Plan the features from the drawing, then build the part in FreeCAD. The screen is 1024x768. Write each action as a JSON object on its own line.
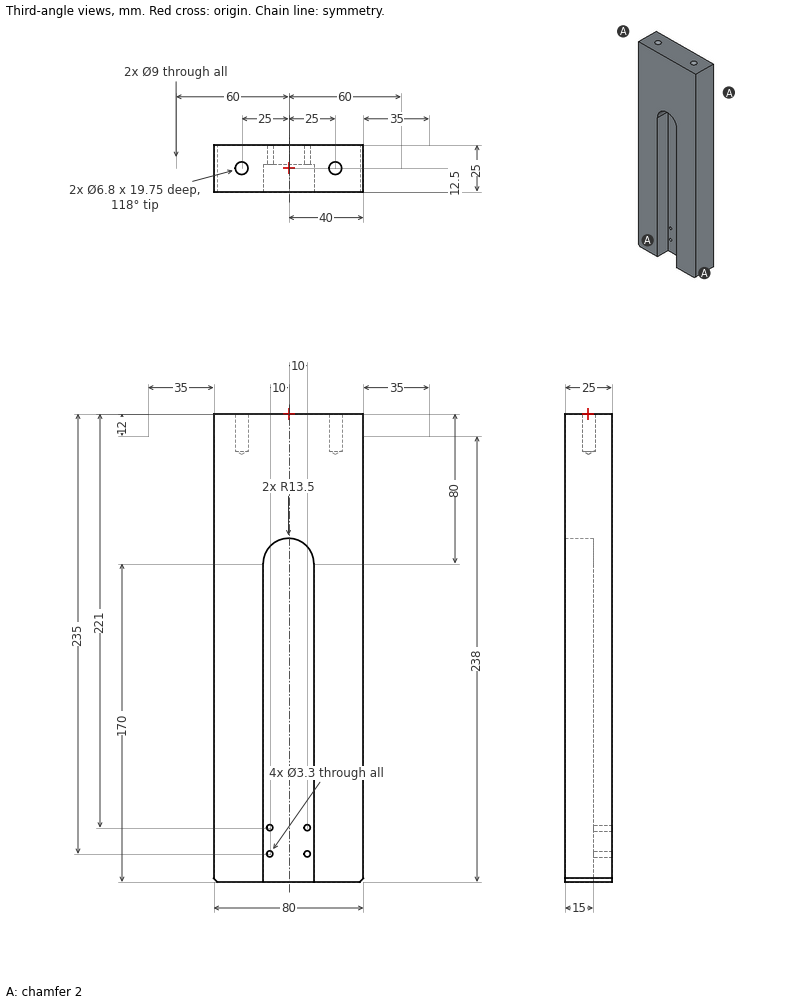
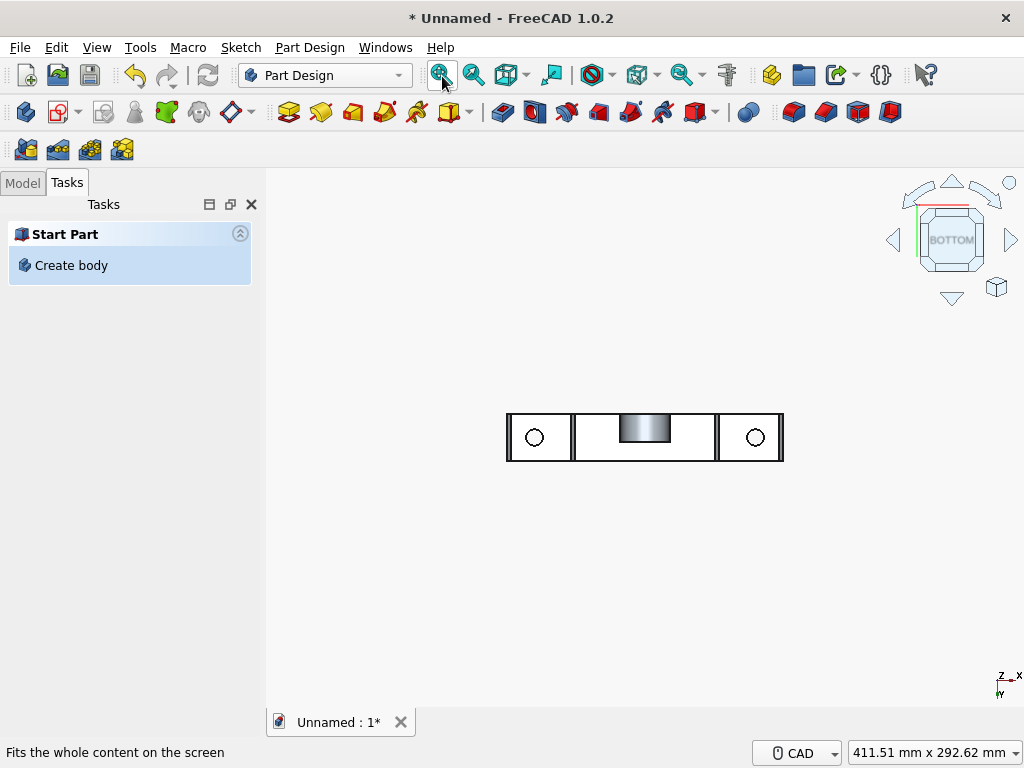
{"action": "left_click", "coordinate": [732, 443]}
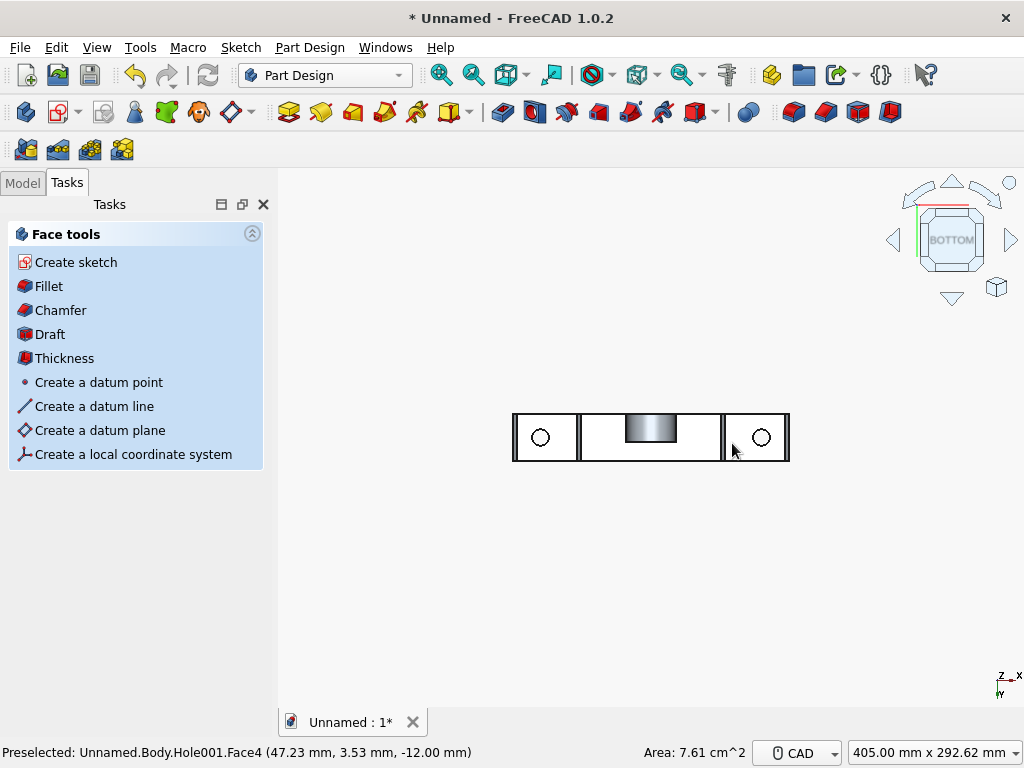
{"action": "left_click", "coordinate": [58, 112]}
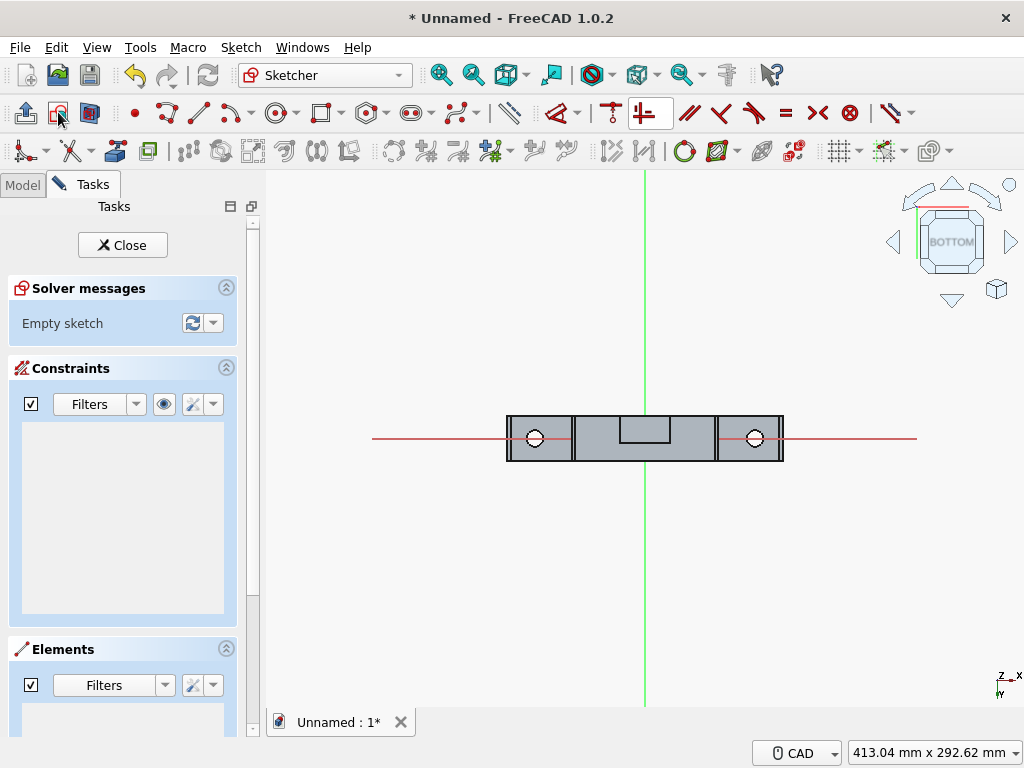
{"action": "scroll", "coordinate": [784, 438], "scroll_direction": "up", "scroll_amount": 2}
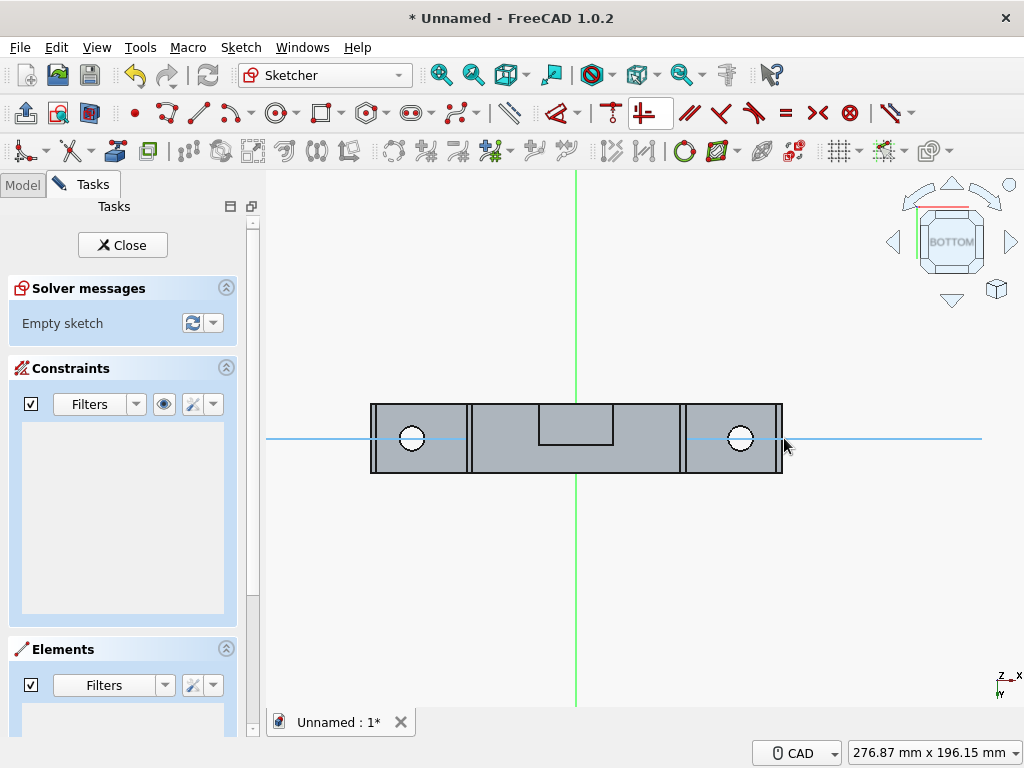
{"action": "key", "text": "g r"}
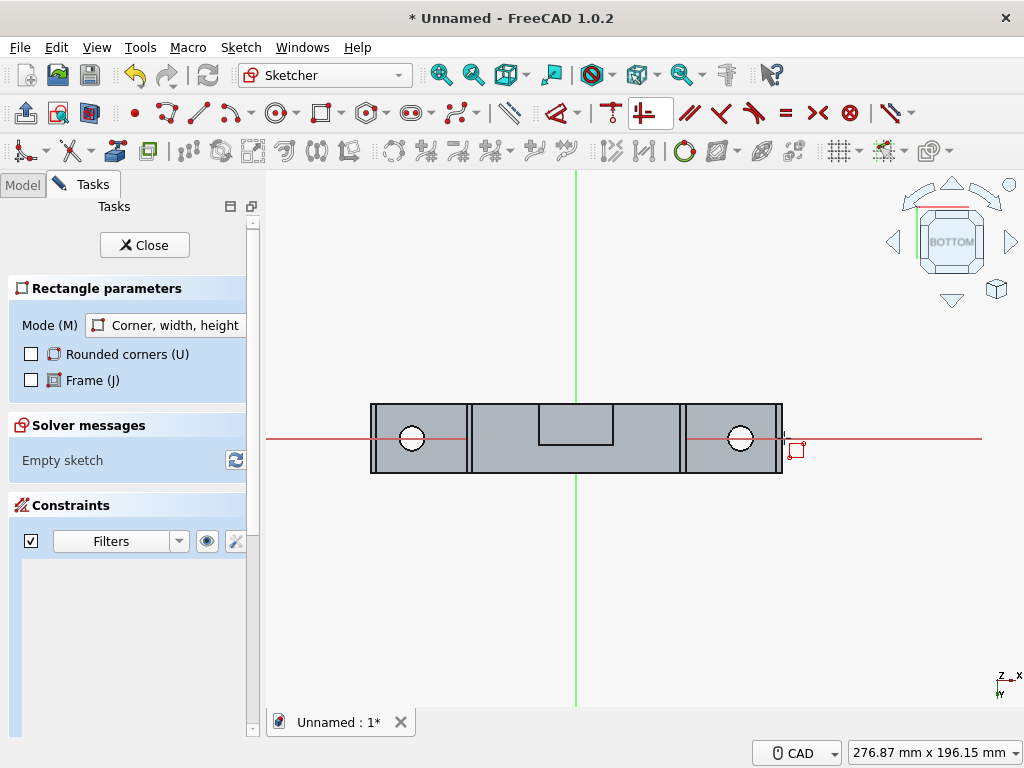
{"action": "left_click", "coordinate": [686, 404]}
{"action": "left_click", "coordinate": [782, 473]}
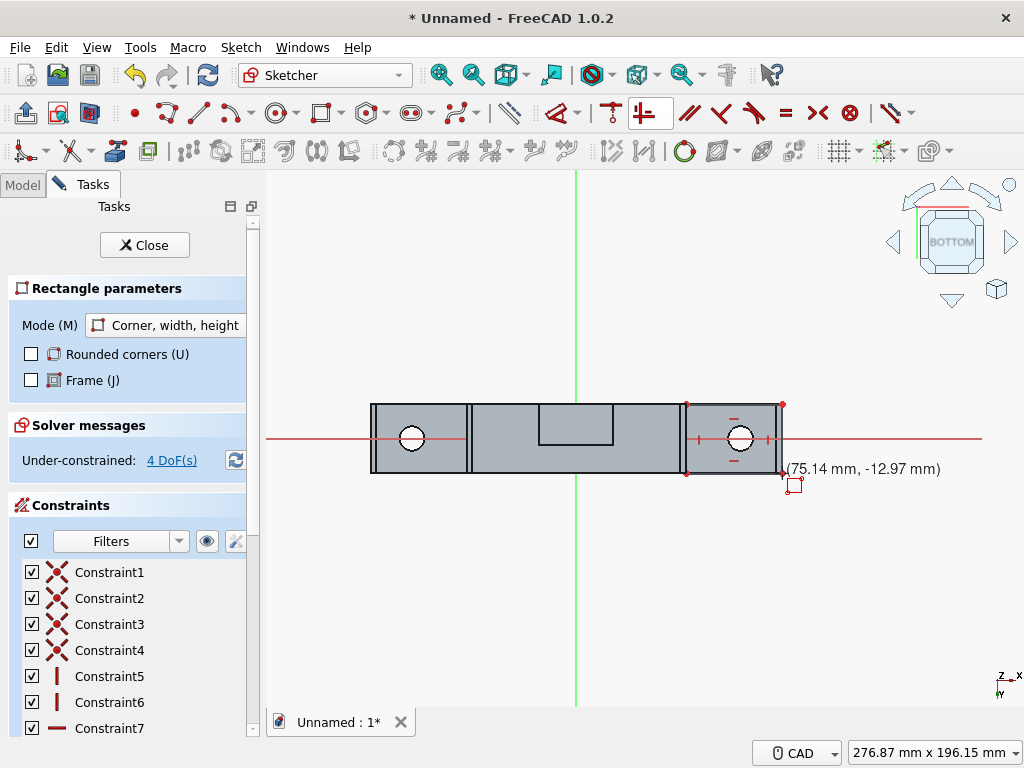
{"action": "left_click", "coordinate": [371, 404]}
{"action": "left_click", "coordinate": [467, 473]}
{"action": "key", "text": "Escape"}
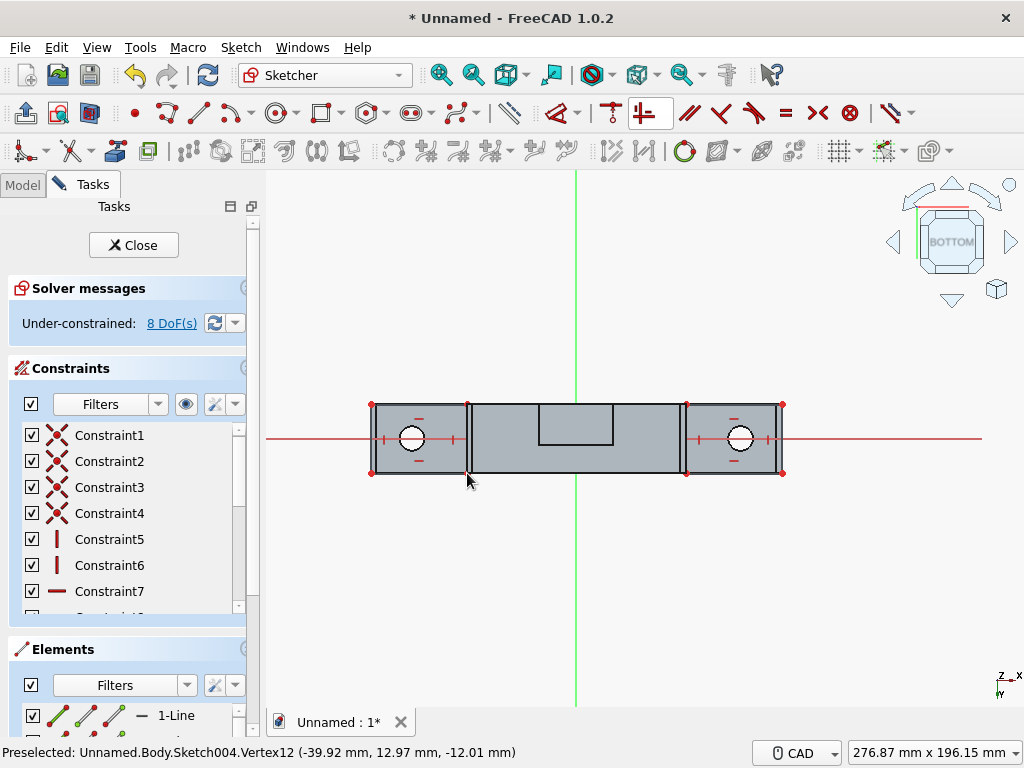
{"action": "left_click", "coordinate": [782, 405]}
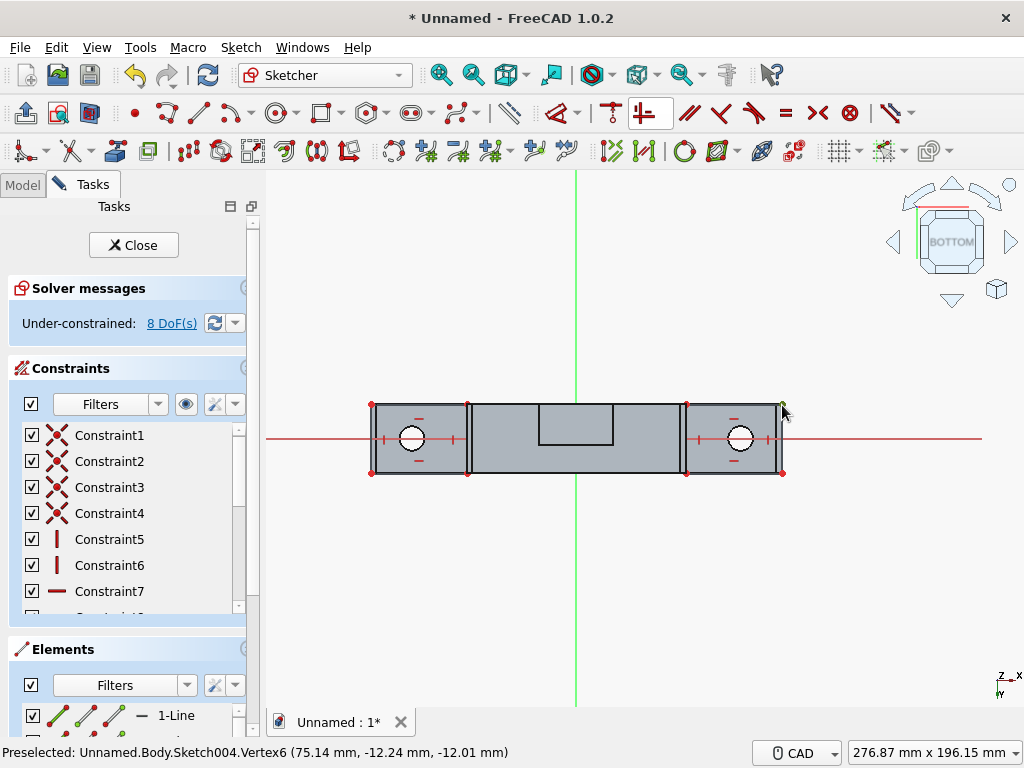
{"action": "left_click", "coordinate": [371, 405]}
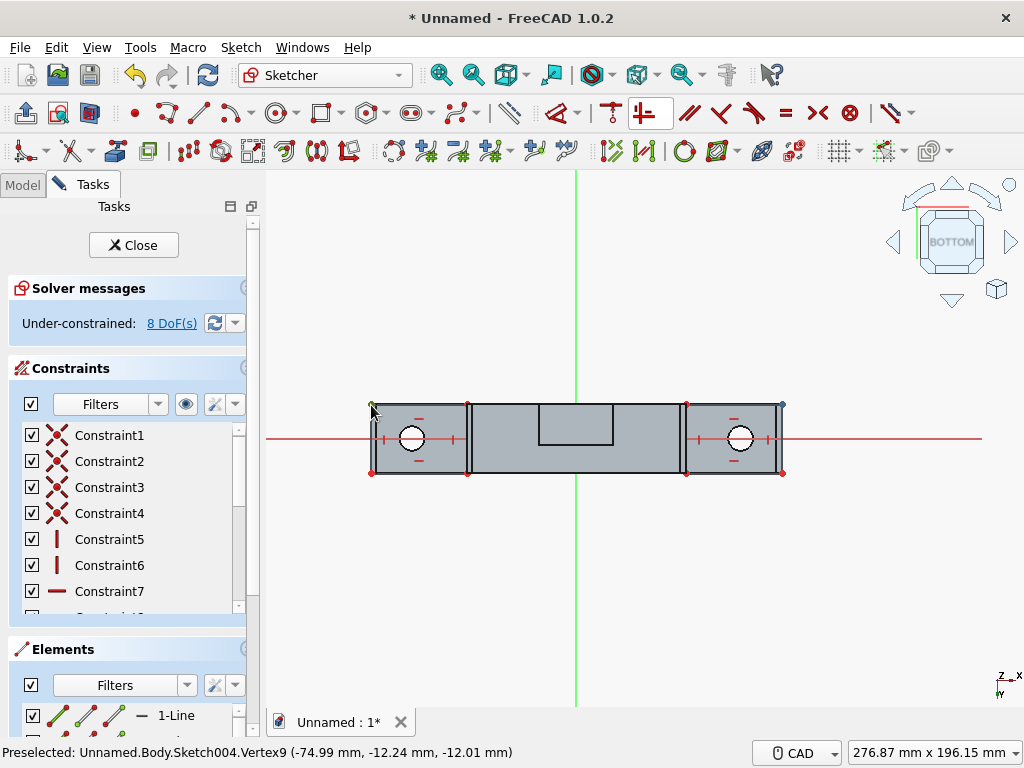
{"action": "left_click", "coordinate": [576, 645]}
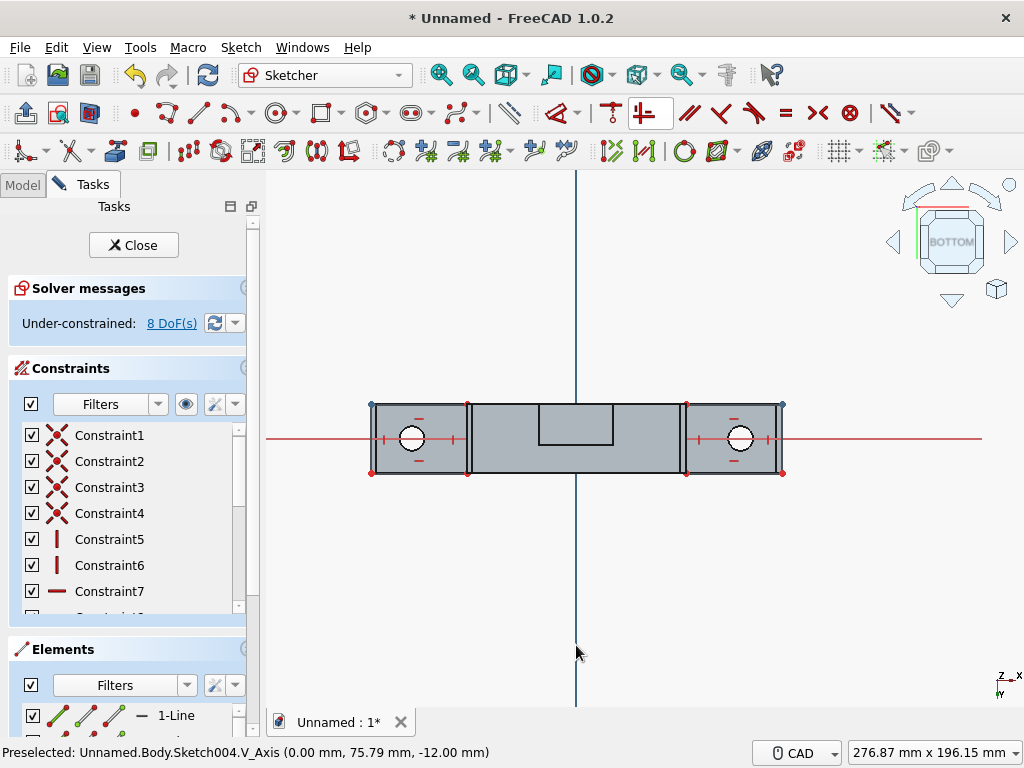
{"action": "left_click", "coordinate": [818, 114]}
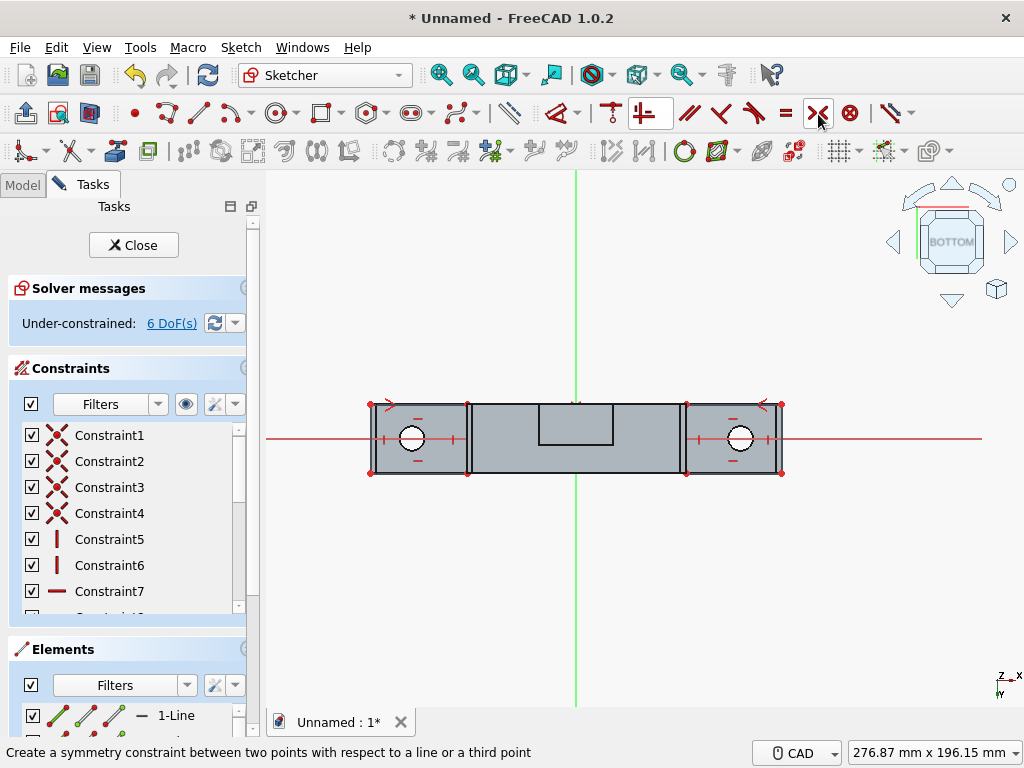
{"action": "left_click", "coordinate": [686, 474]}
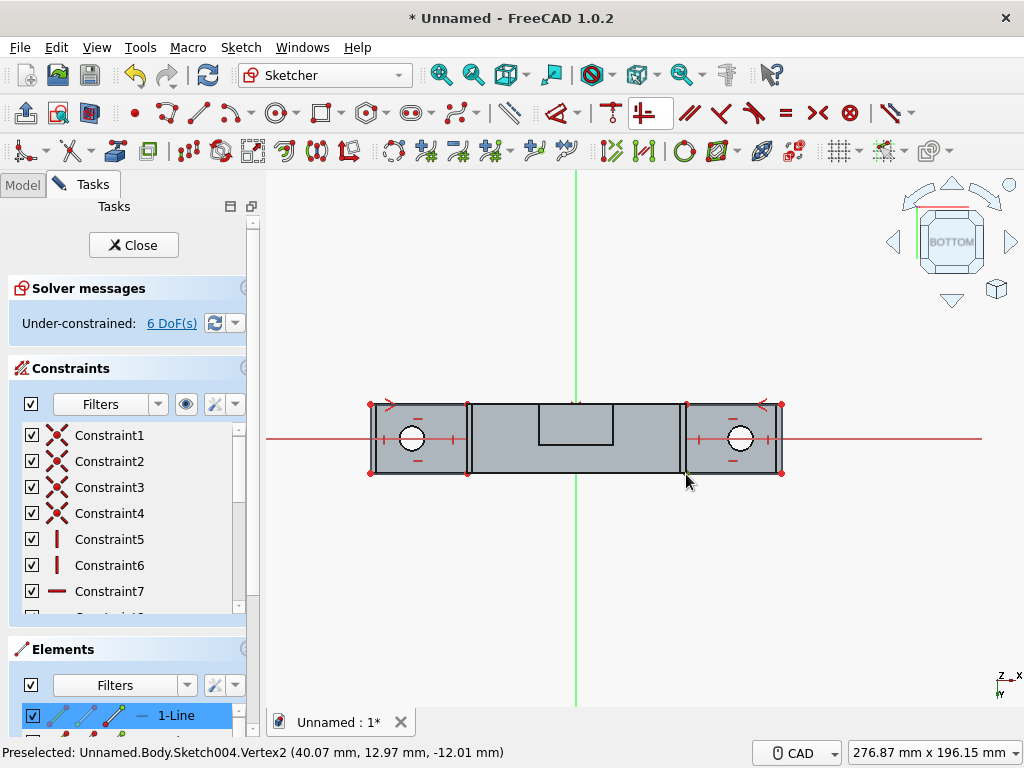
{"action": "left_click", "coordinate": [467, 474]}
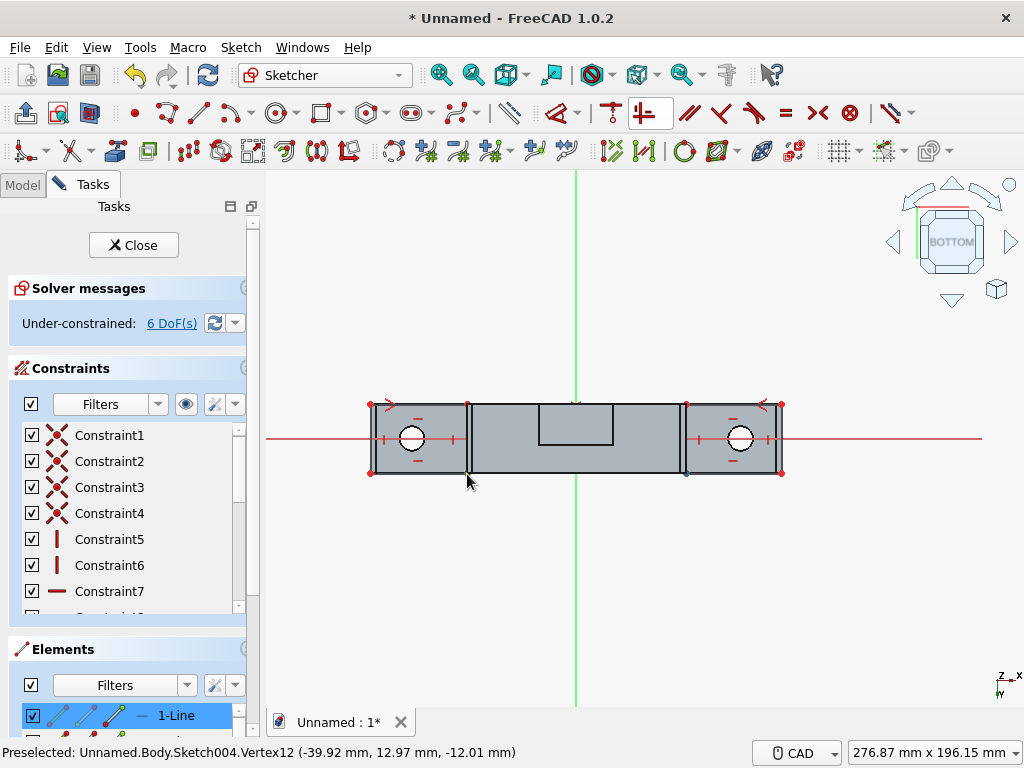
{"action": "left_click", "coordinate": [576, 645]}